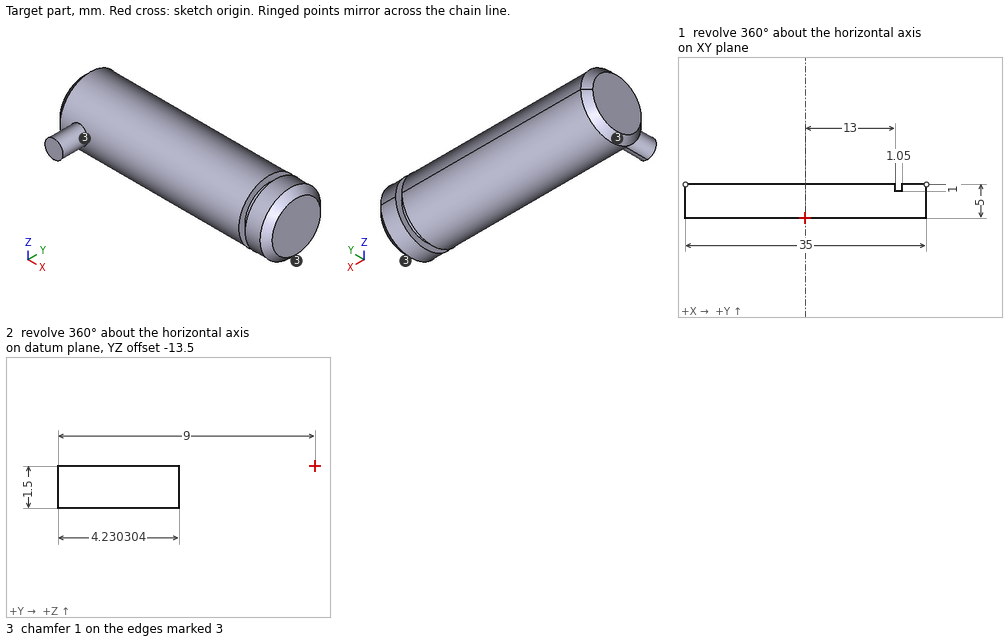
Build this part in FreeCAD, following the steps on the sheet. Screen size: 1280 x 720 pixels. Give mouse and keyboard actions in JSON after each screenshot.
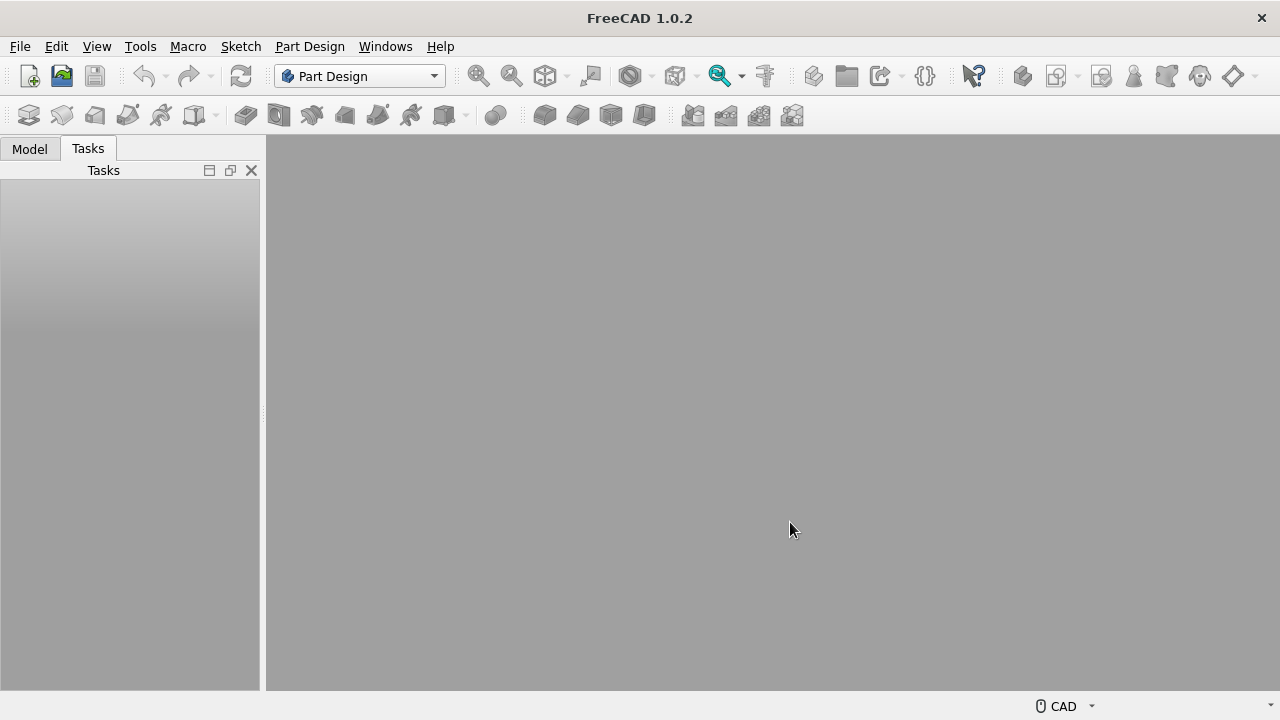
{"action": "left_click", "coordinate": [29, 76]}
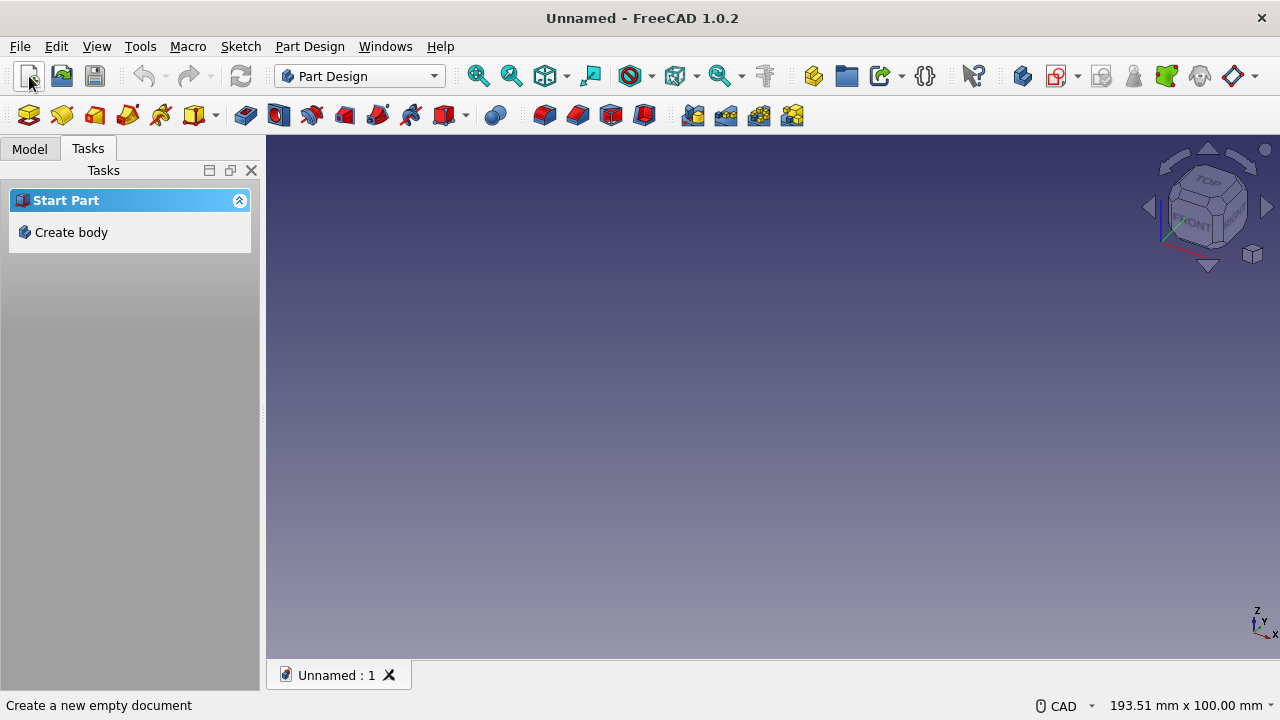
{"action": "left_click", "coordinate": [1056, 76]}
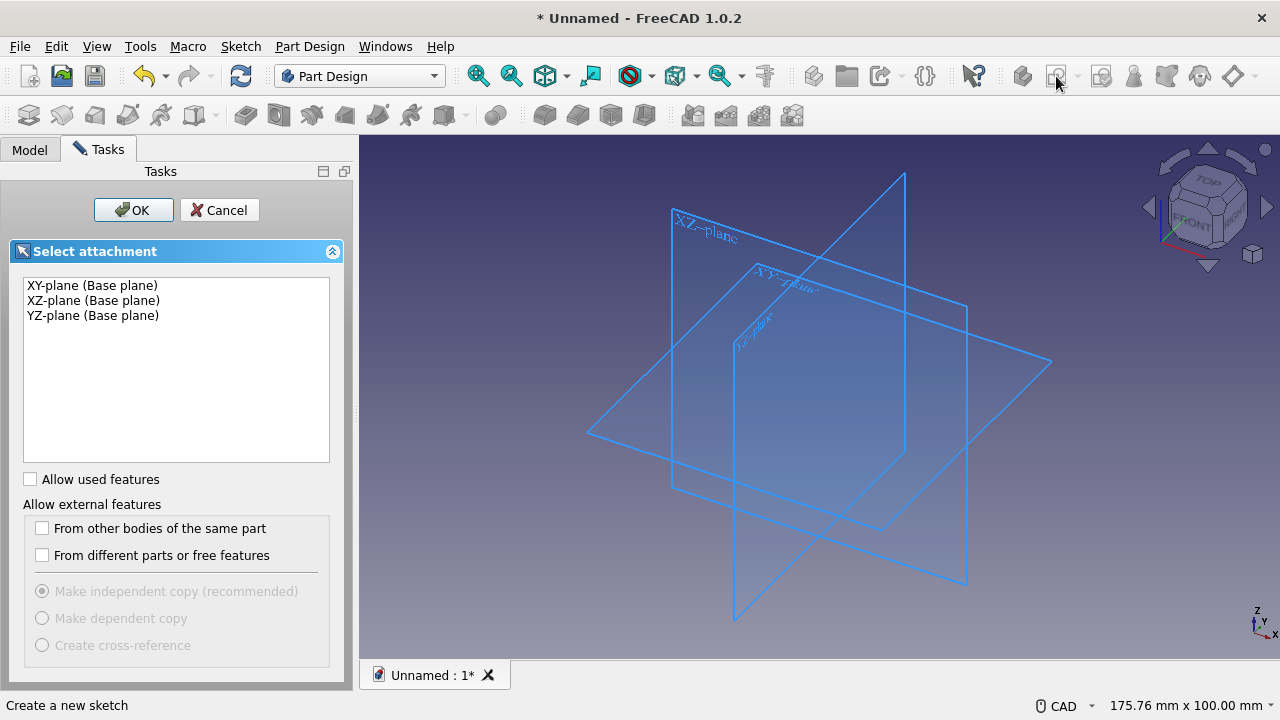
{"action": "left_click", "coordinate": [84, 286]}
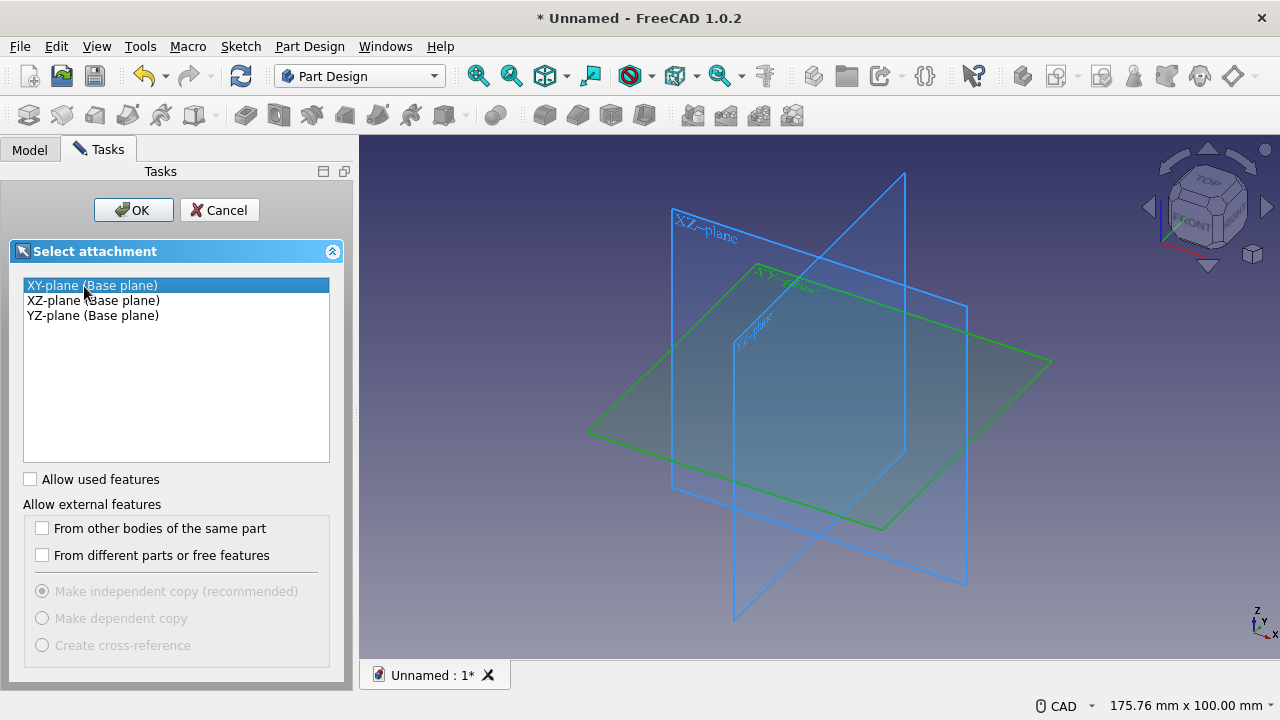
{"action": "left_click", "coordinate": [134, 210]}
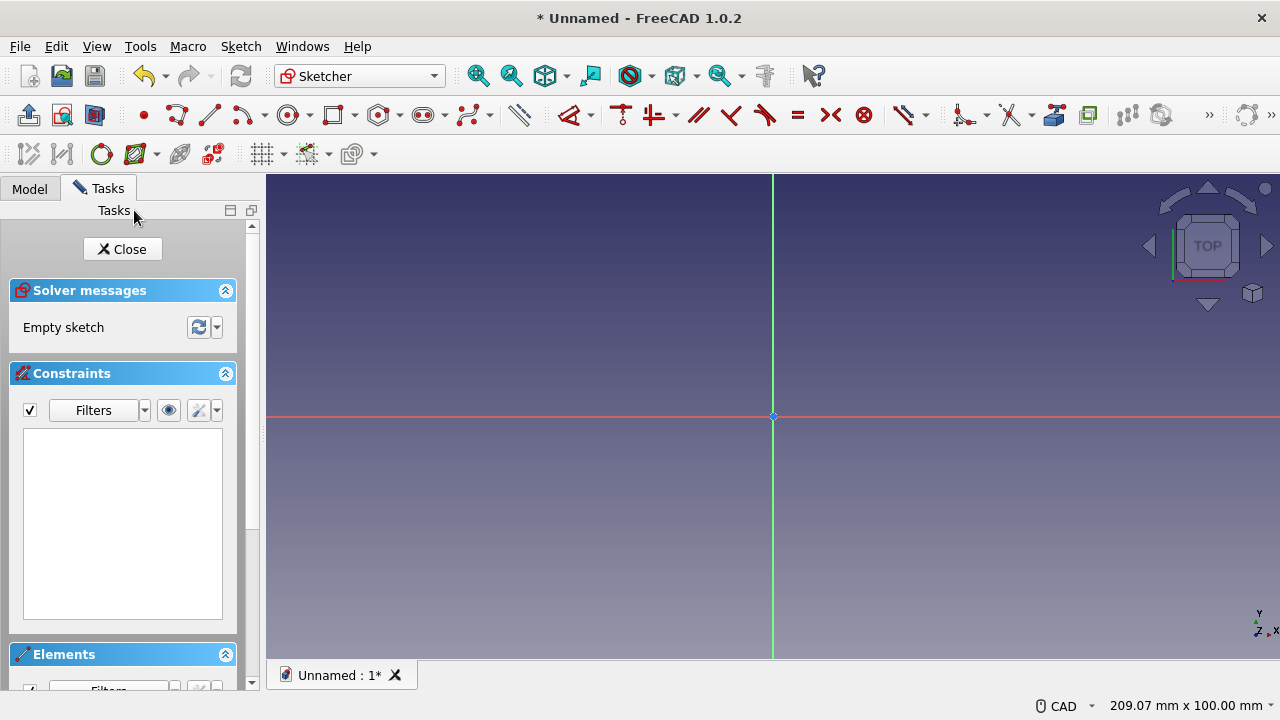
{"action": "scroll", "coordinate": [803, 399], "scroll_direction": "up", "scroll_amount": 6}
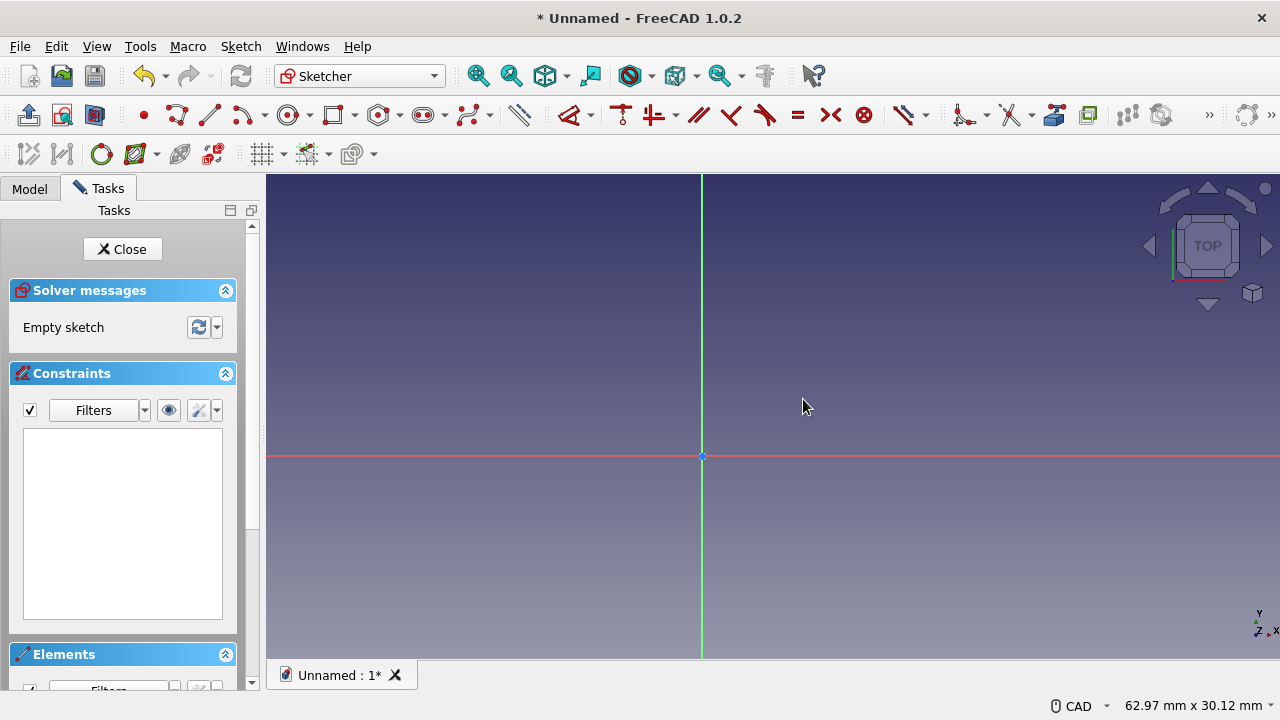
{"action": "left_click", "coordinate": [177, 116]}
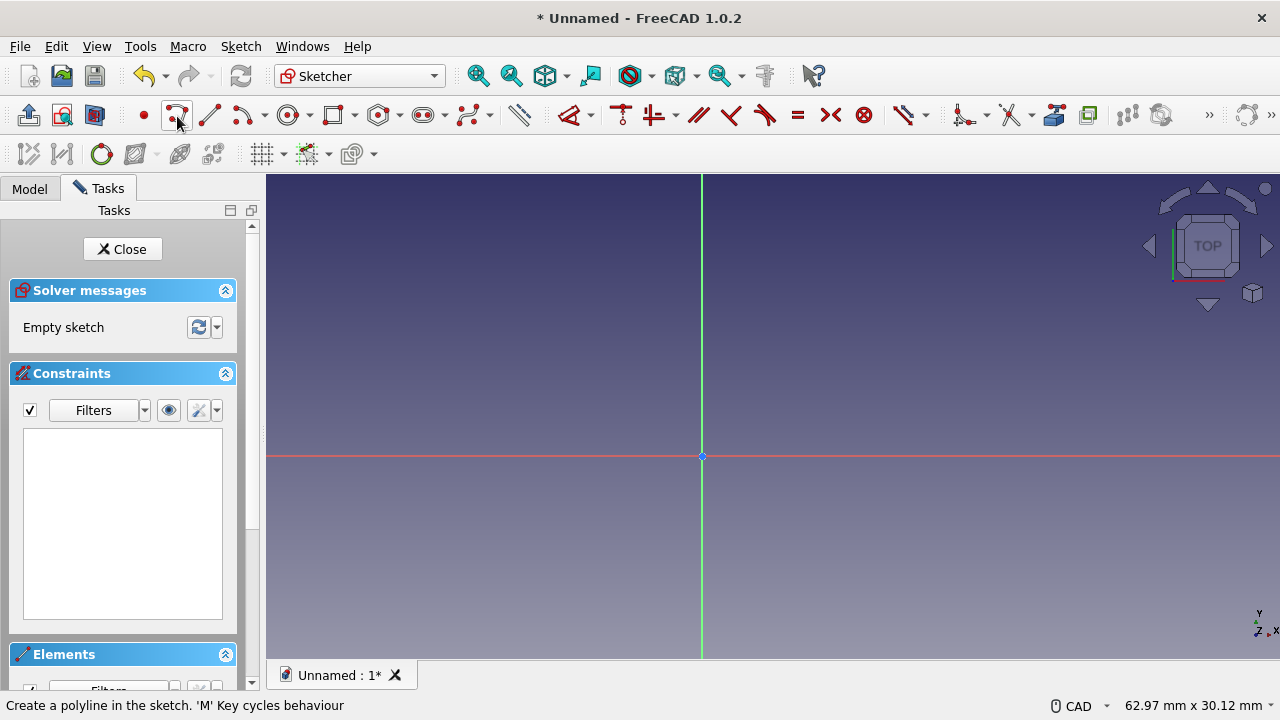
{"action": "left_click", "coordinate": [911, 392]}
{"action": "left_click", "coordinate": [928, 392]}
{"action": "left_click", "coordinate": [928, 376]}
{"action": "left_click", "coordinate": [984, 376]}
{"action": "left_click", "coordinate": [984, 456]}
{"action": "left_click", "coordinate": [420, 447]}
{"action": "left_click", "coordinate": [420, 376]}
{"action": "left_click", "coordinate": [911, 376]}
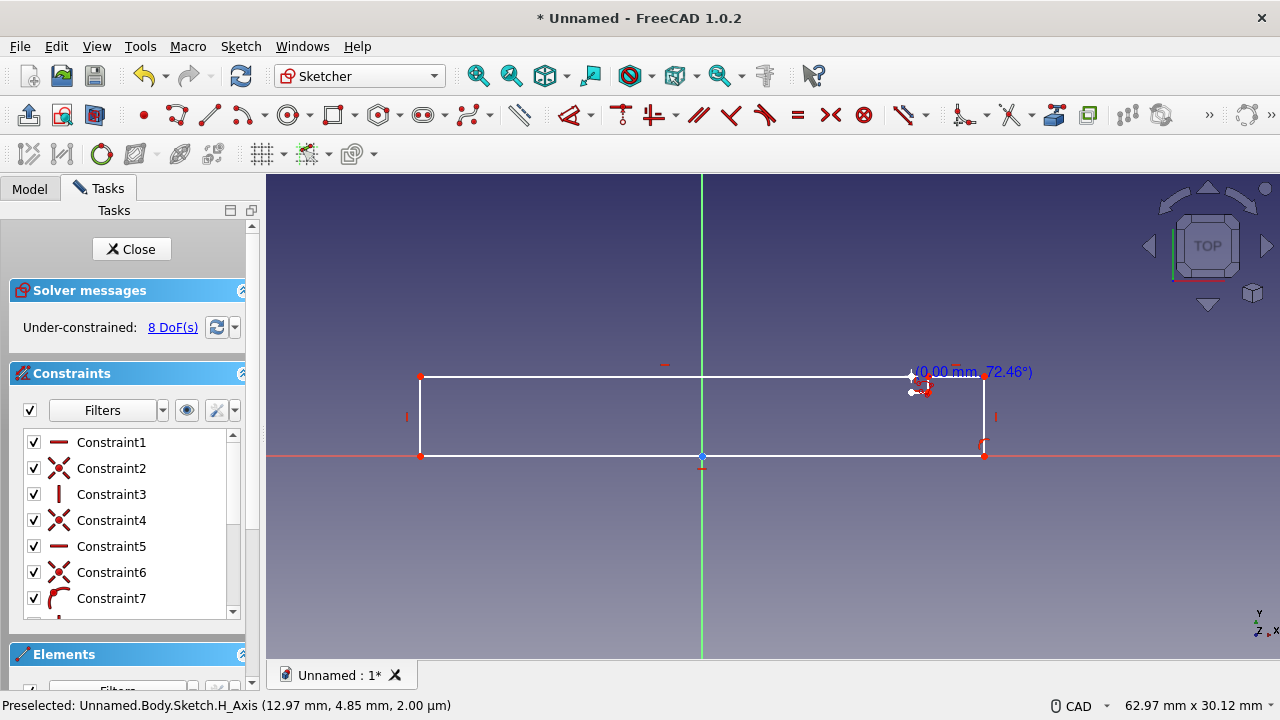
{"action": "scroll", "coordinate": [911, 392], "scroll_direction": "up", "scroll_amount": 4}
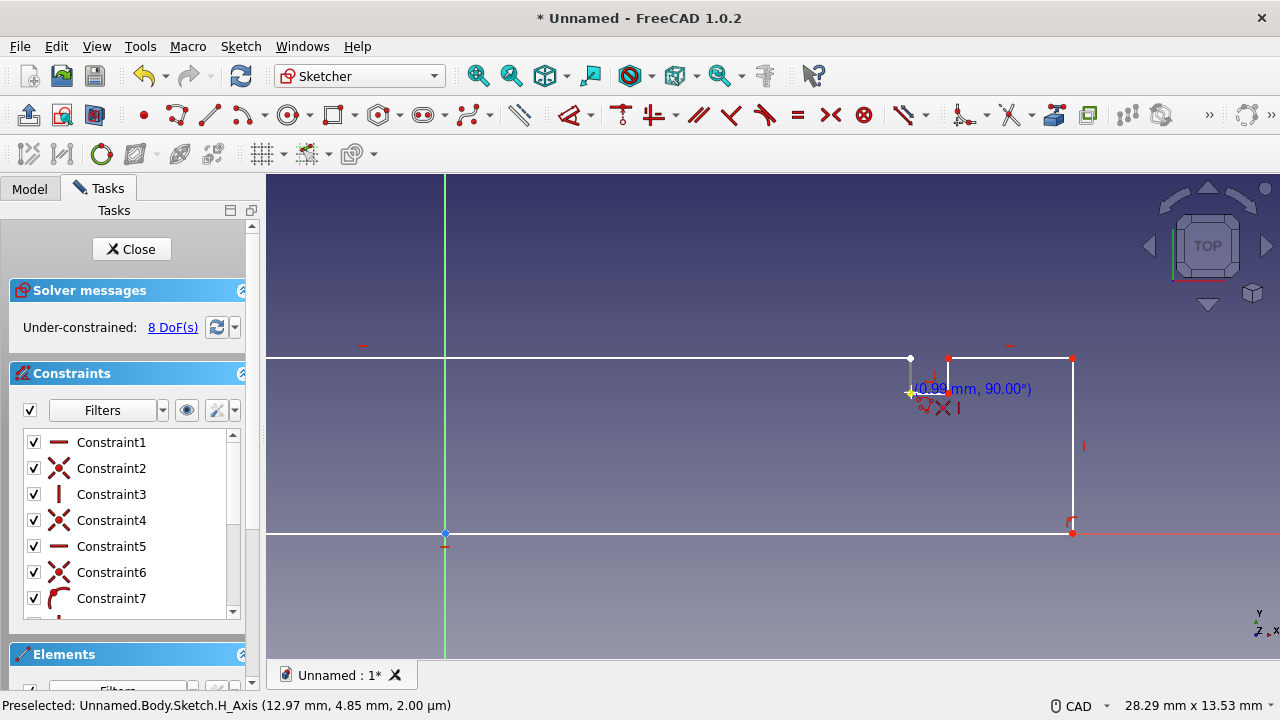
{"action": "left_click", "coordinate": [910, 394]}
{"action": "key", "text": "Escape"}
{"action": "key", "text": "Escape"}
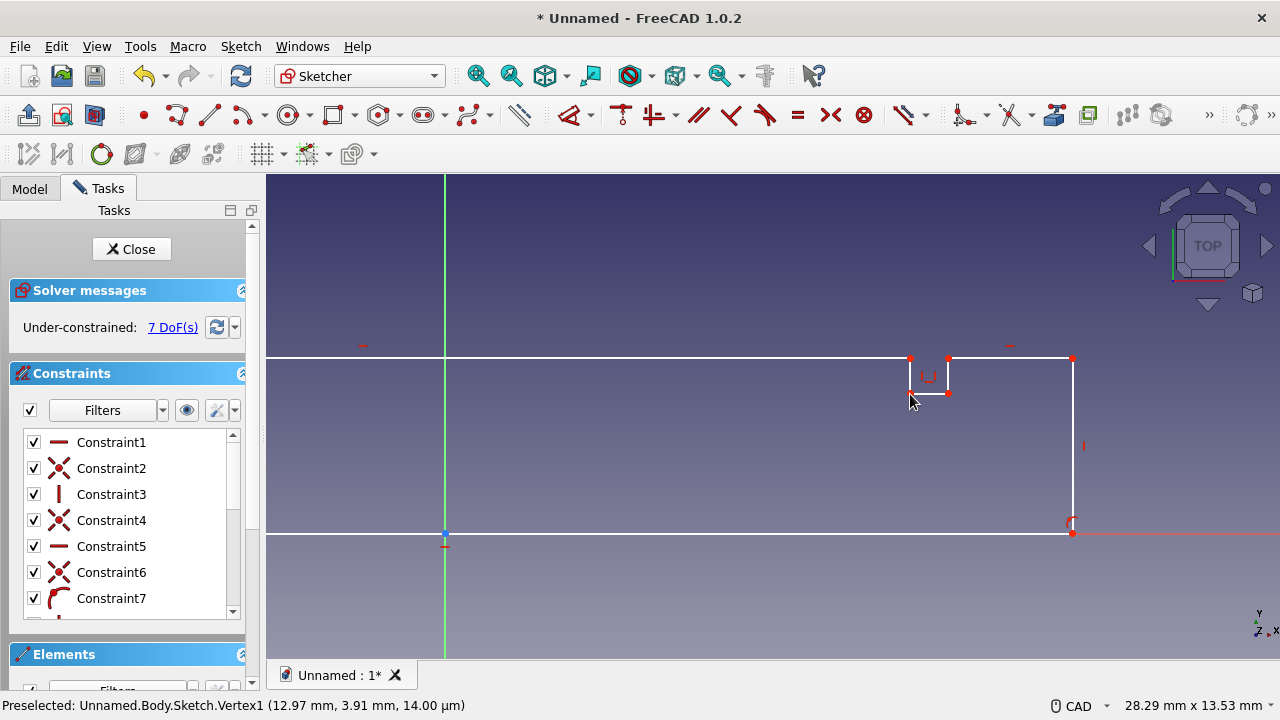
{"action": "left_click", "coordinate": [1073, 358]}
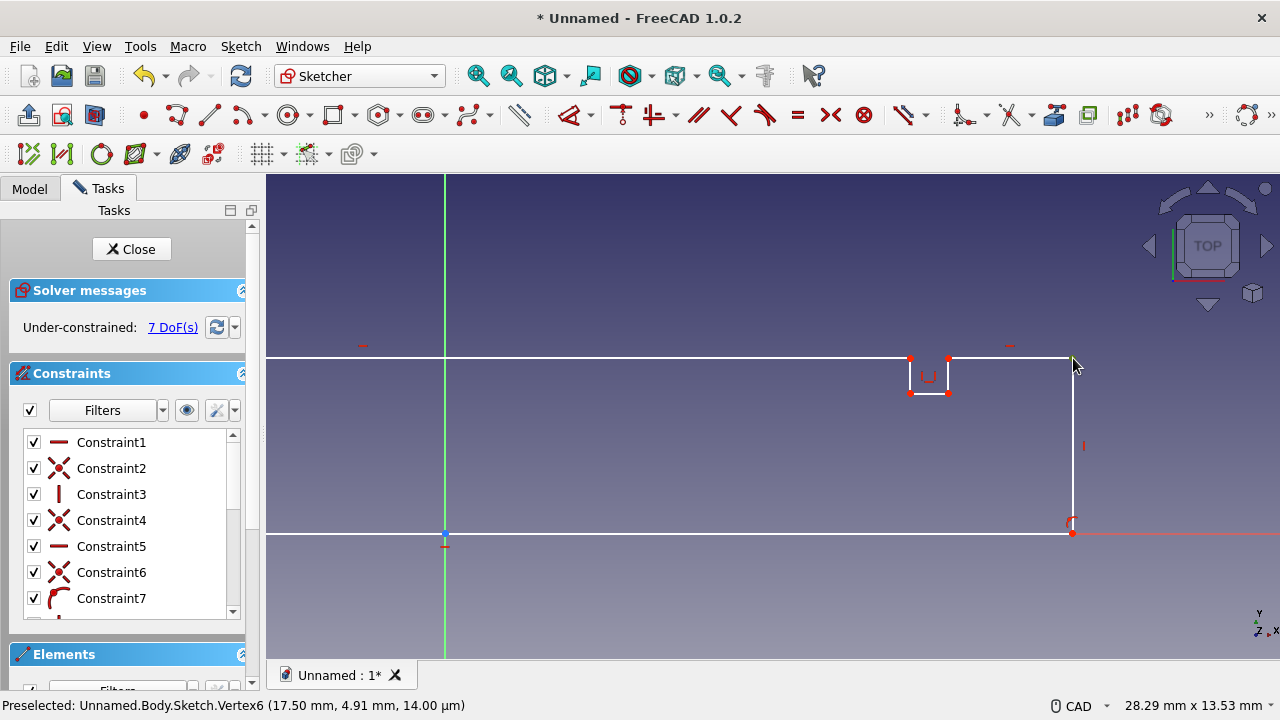
{"action": "scroll", "coordinate": [916, 394], "scroll_direction": "down", "scroll_amount": 4}